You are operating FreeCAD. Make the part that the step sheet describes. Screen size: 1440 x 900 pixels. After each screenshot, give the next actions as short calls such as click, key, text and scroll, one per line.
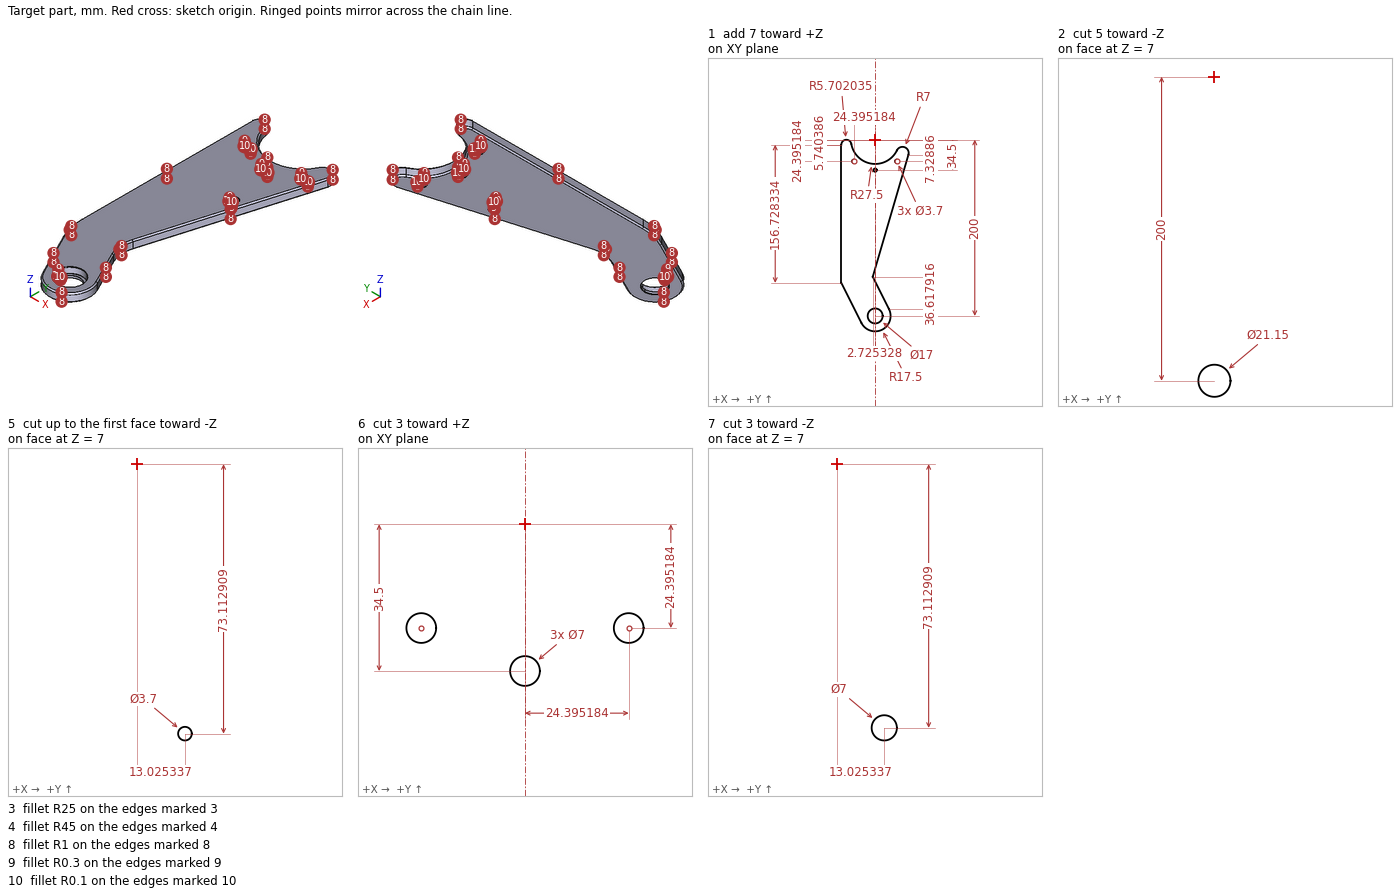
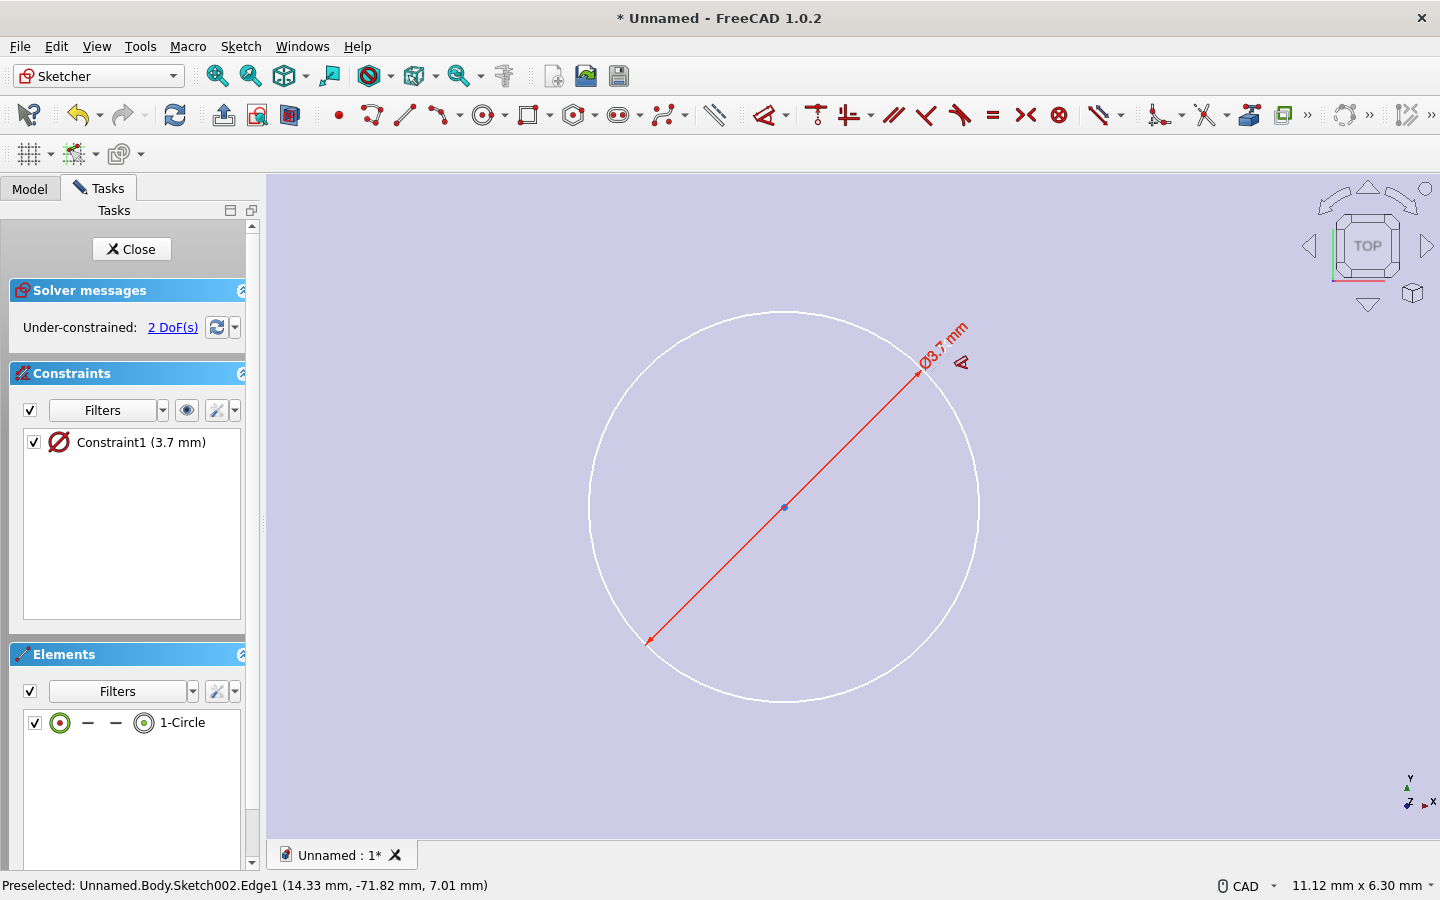
click(784, 507)
click(539, 541)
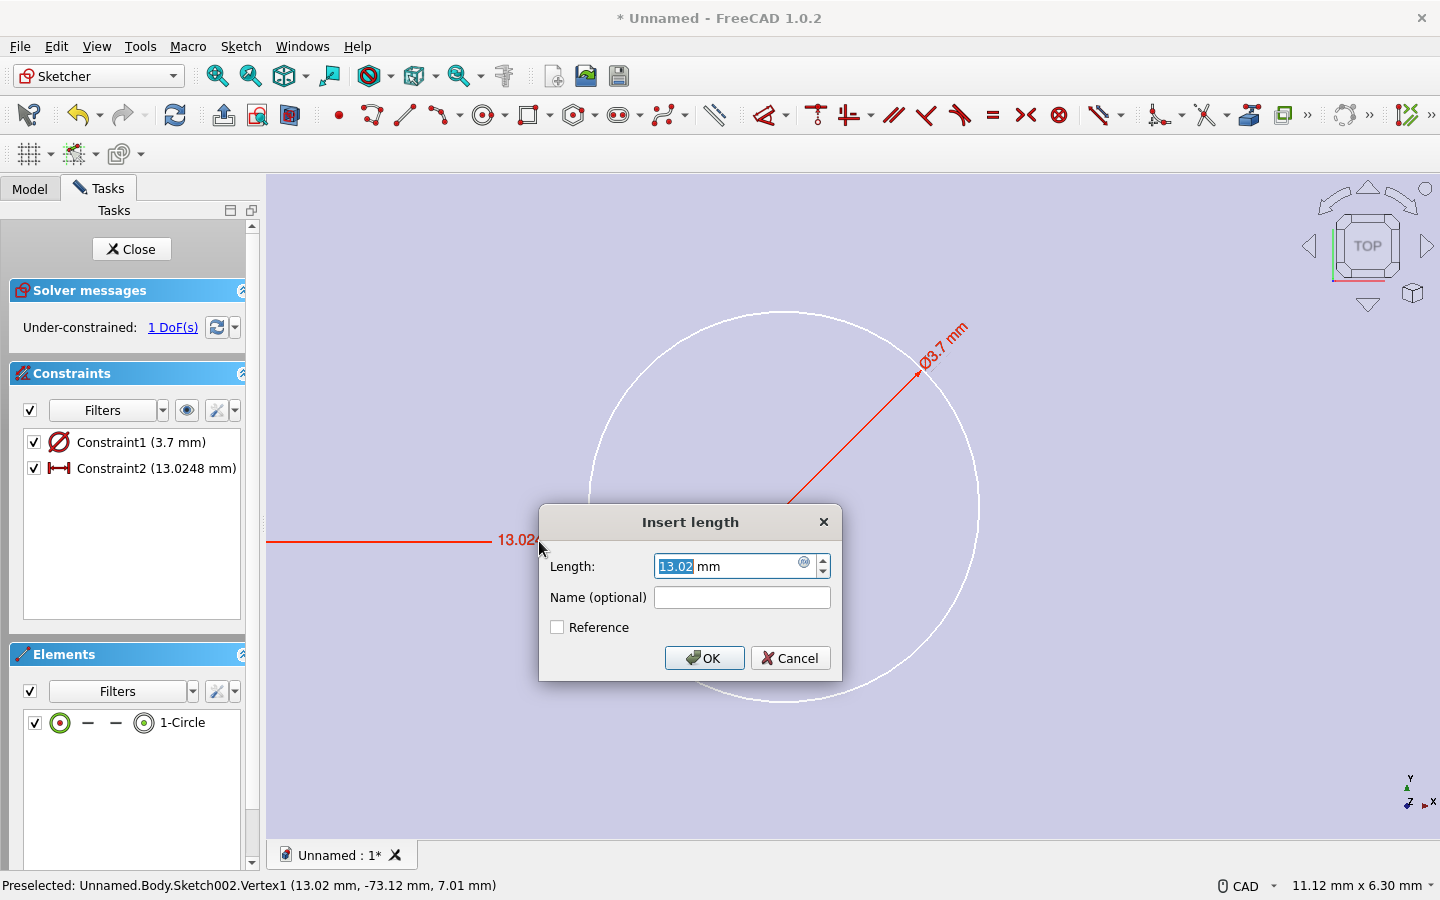
text(13.025337)
key(Return)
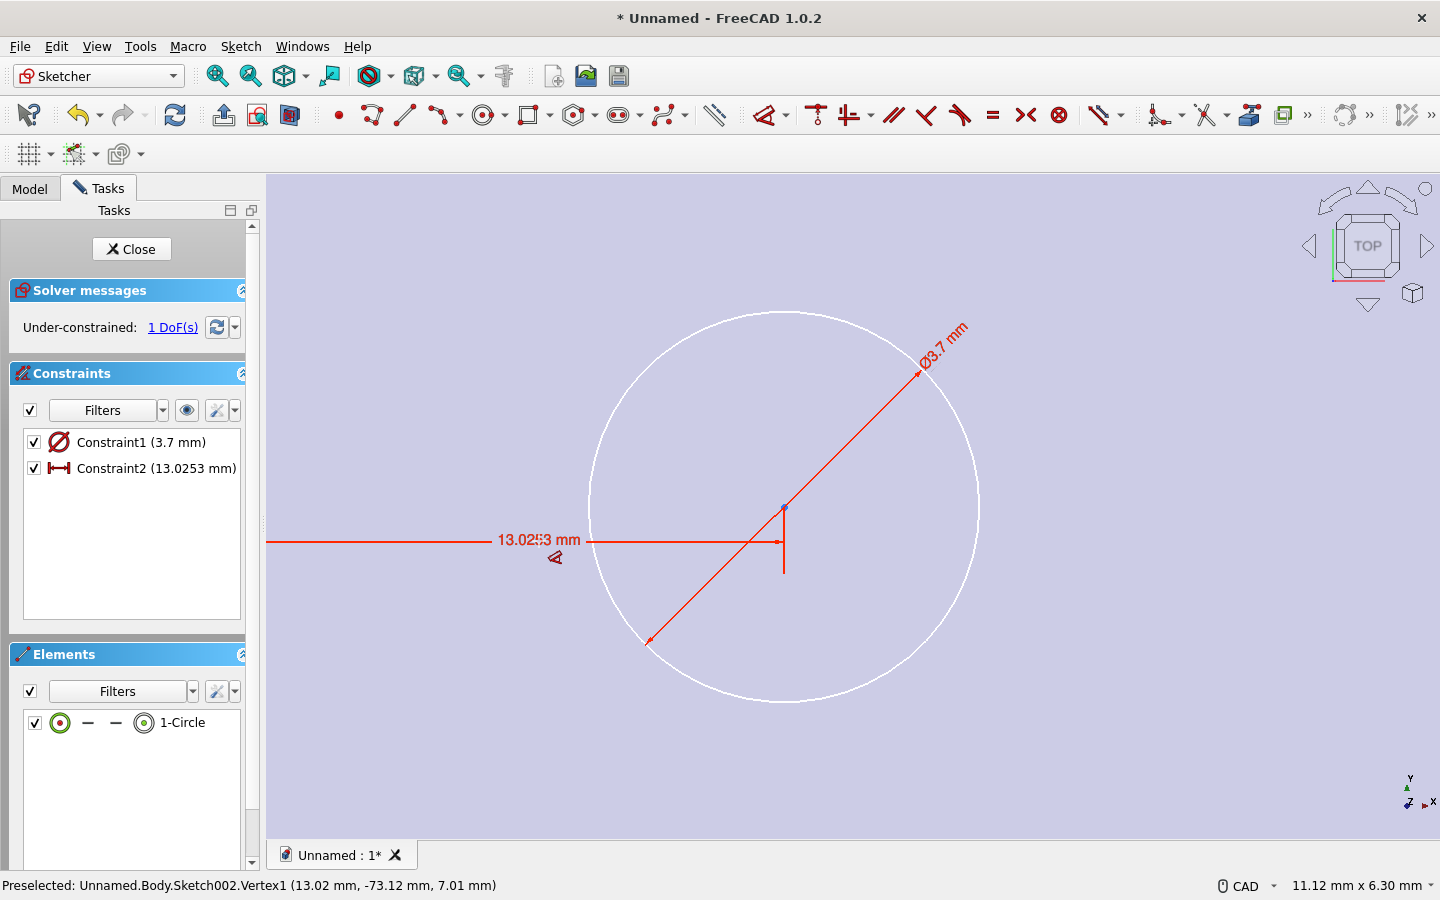
click(784, 507)
click(818, 355)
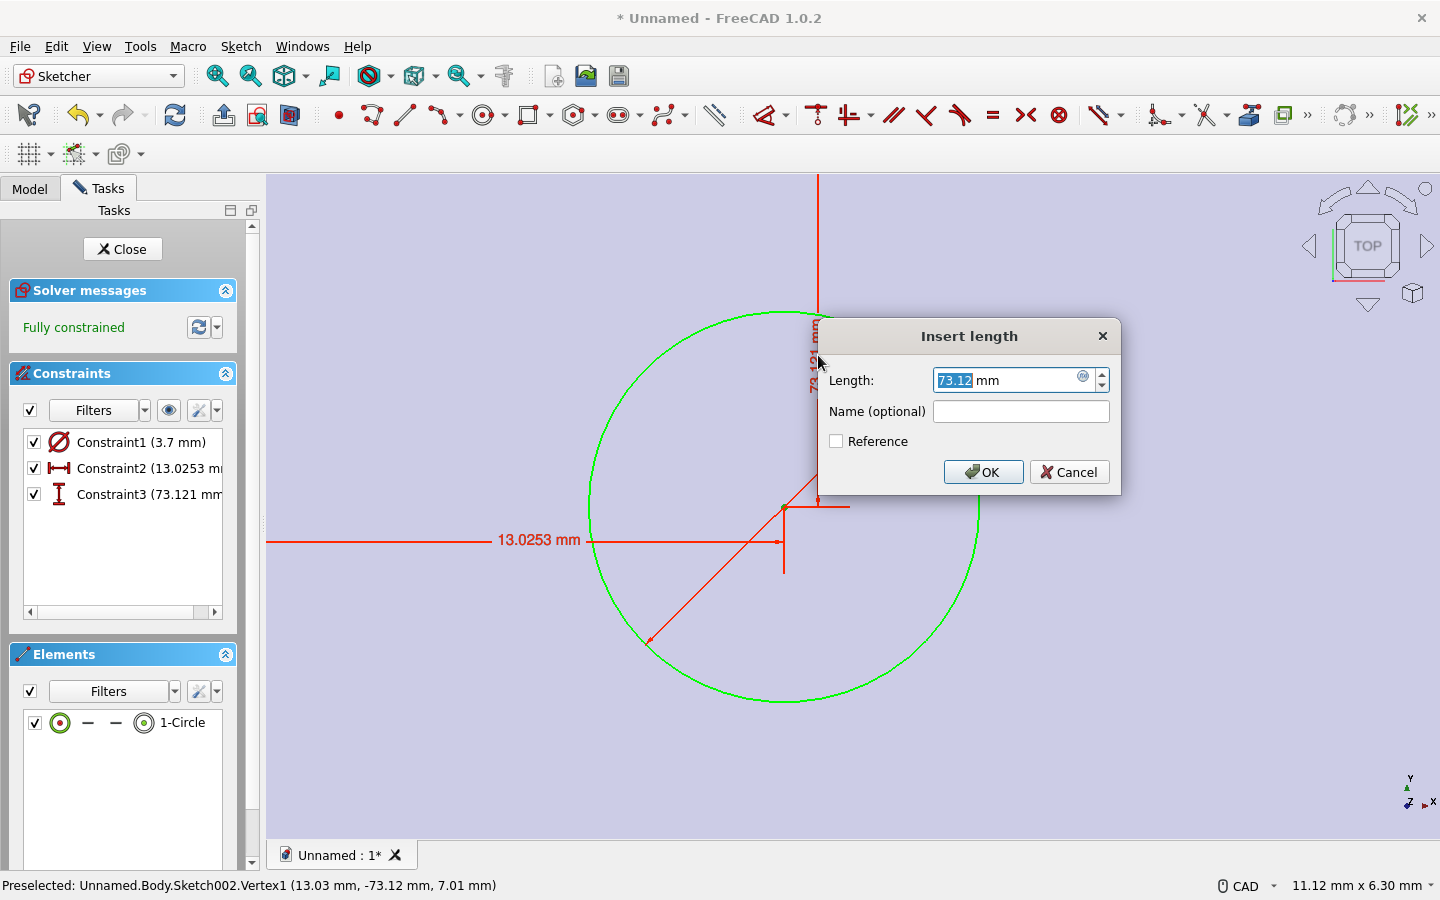
text(73.112909)
key(Return)
key(Escape)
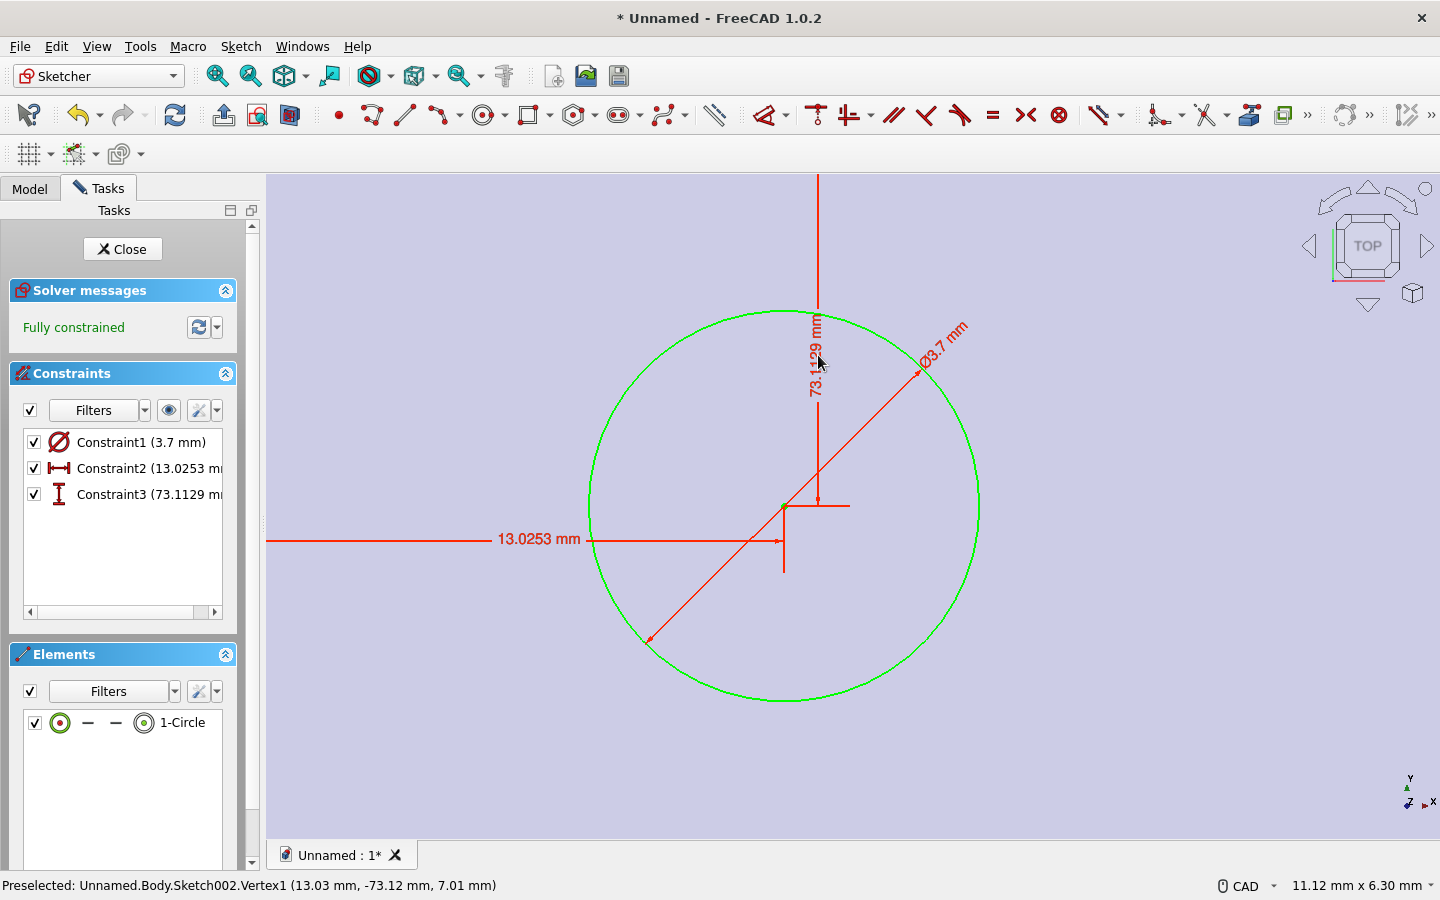
click(123, 249)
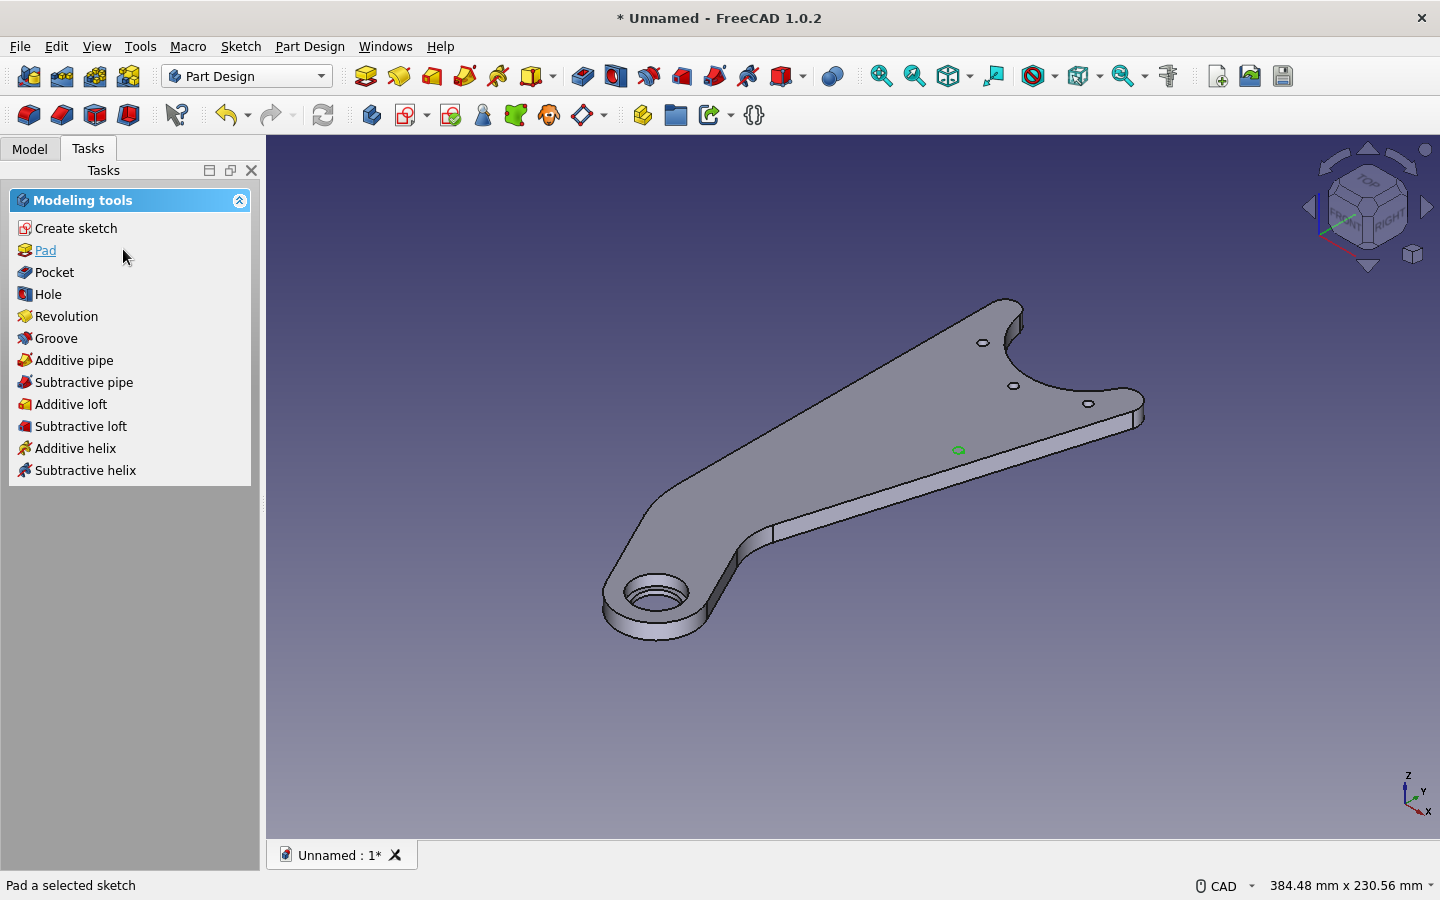
click(583, 76)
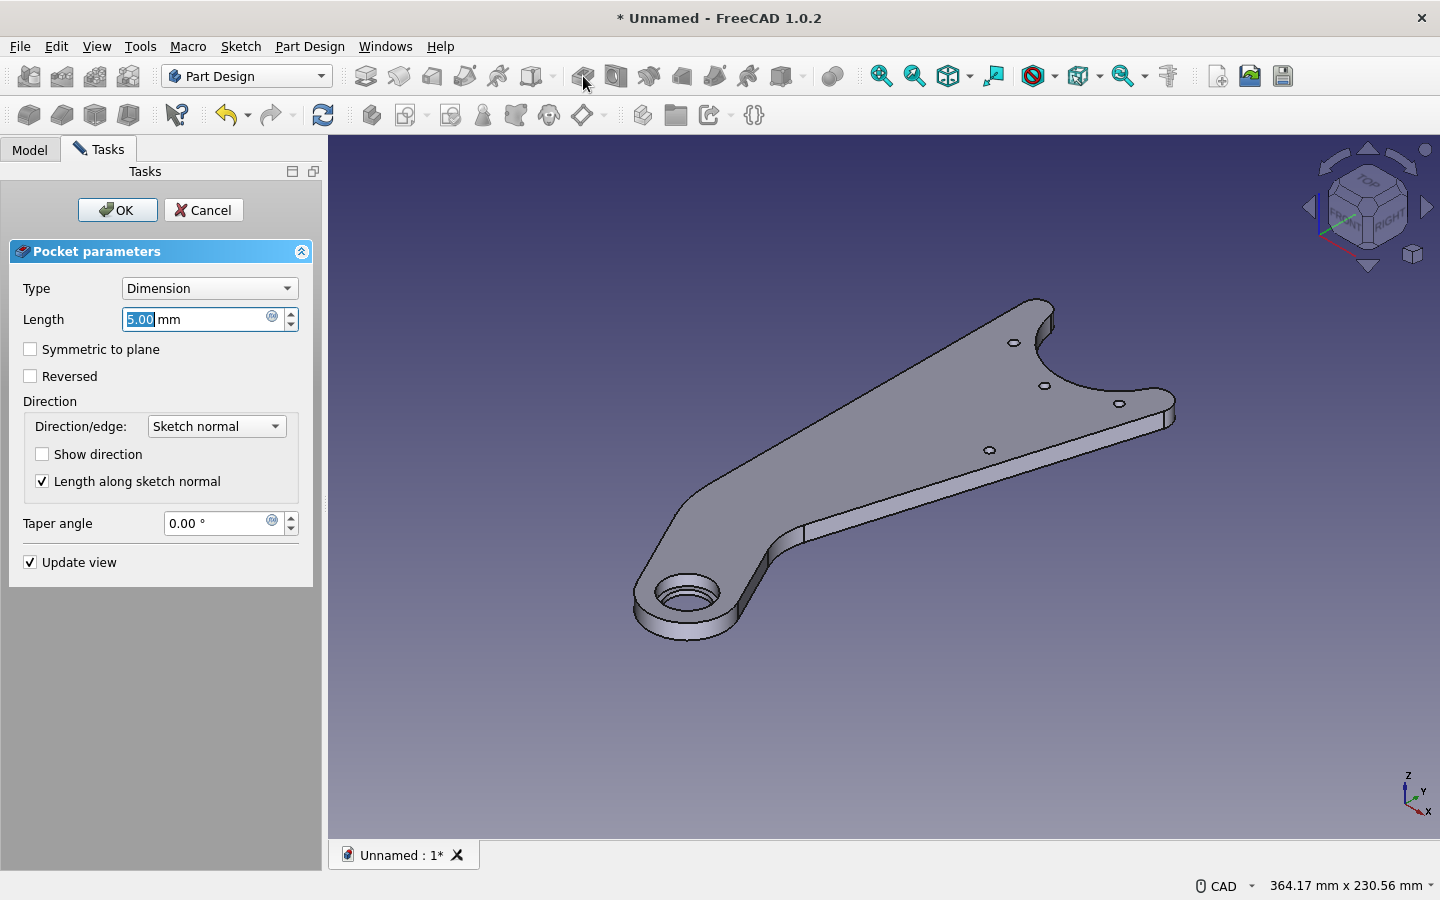
click(210, 288)